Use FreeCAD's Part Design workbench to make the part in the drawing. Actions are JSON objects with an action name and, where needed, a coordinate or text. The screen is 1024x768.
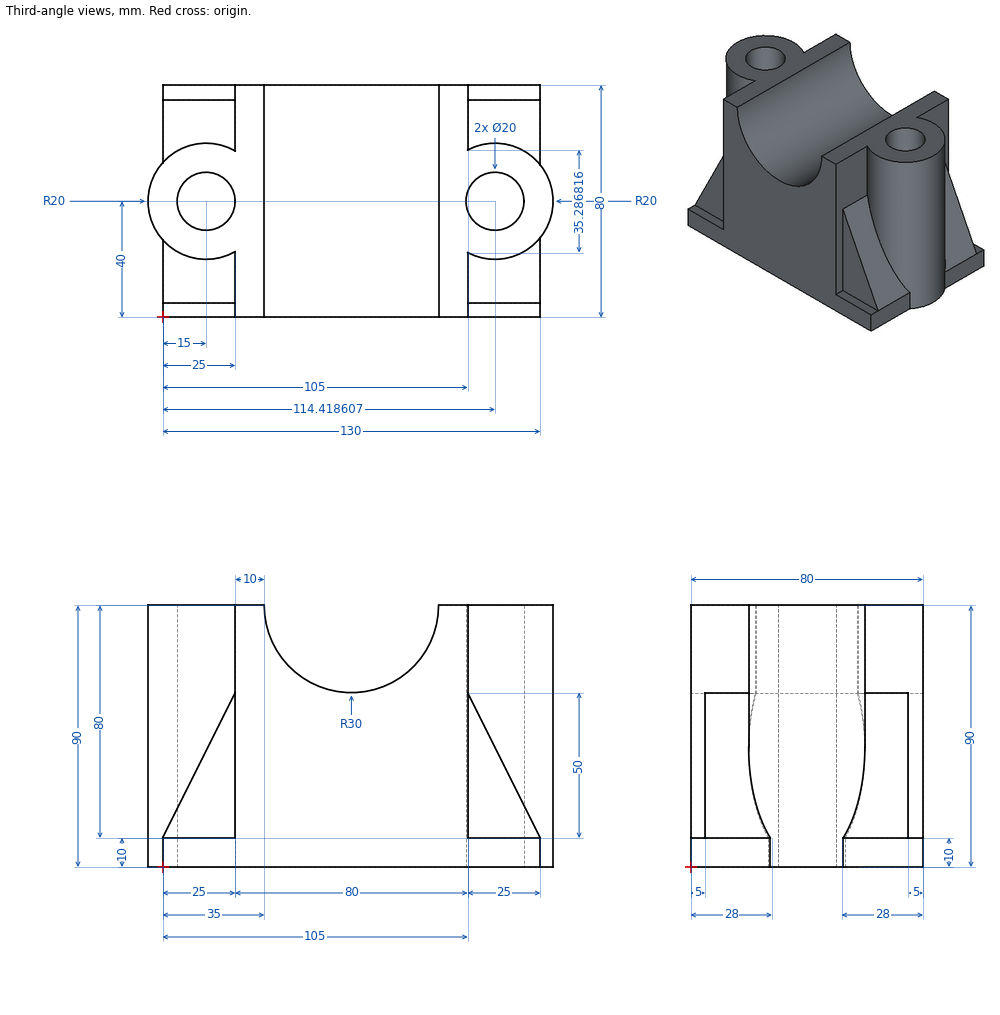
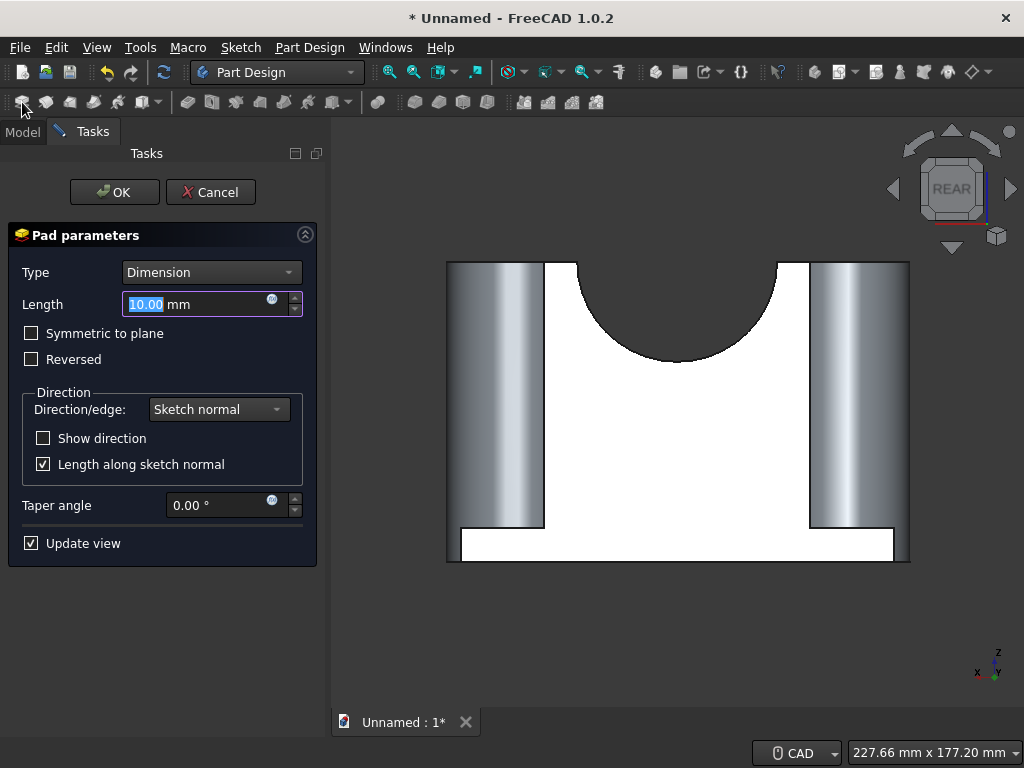
{"action": "type", "text": "28"}
{"action": "key", "text": "Tab"}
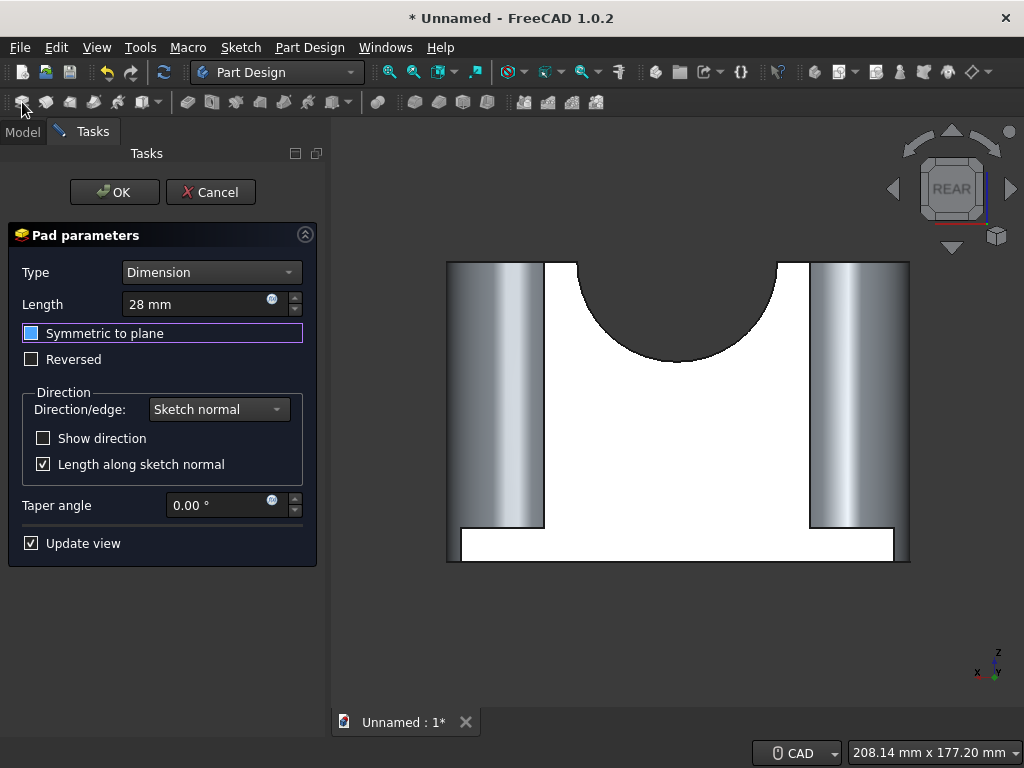
{"action": "left_click", "coordinate": [30, 359]}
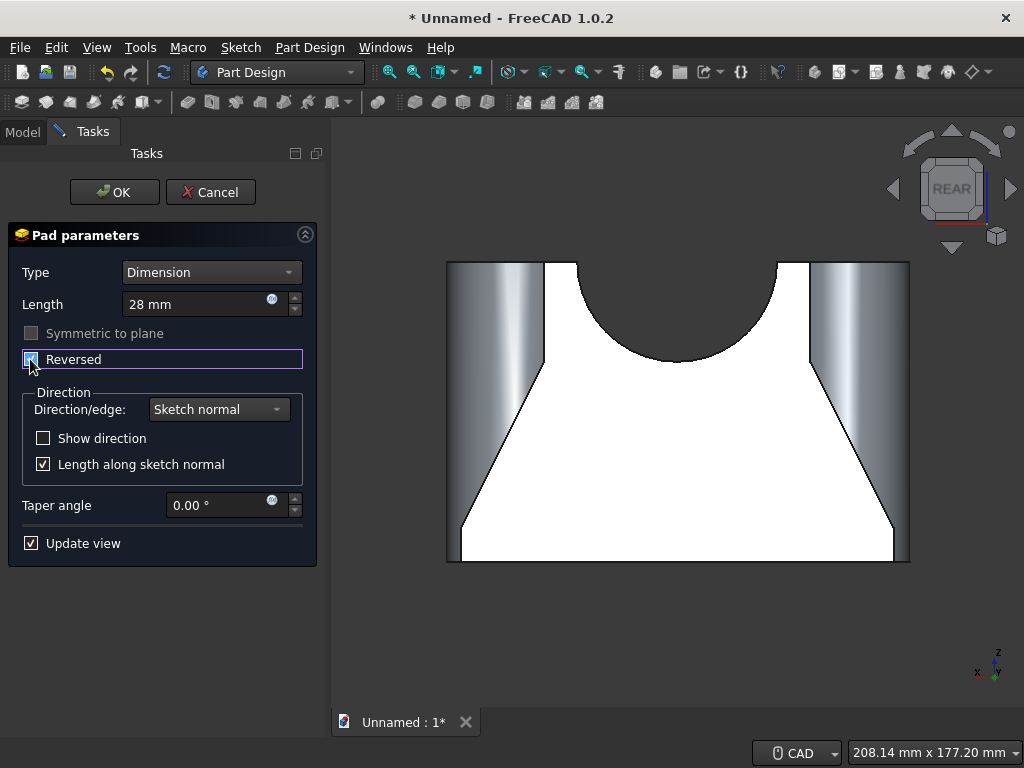
{"action": "left_click", "coordinate": [115, 192]}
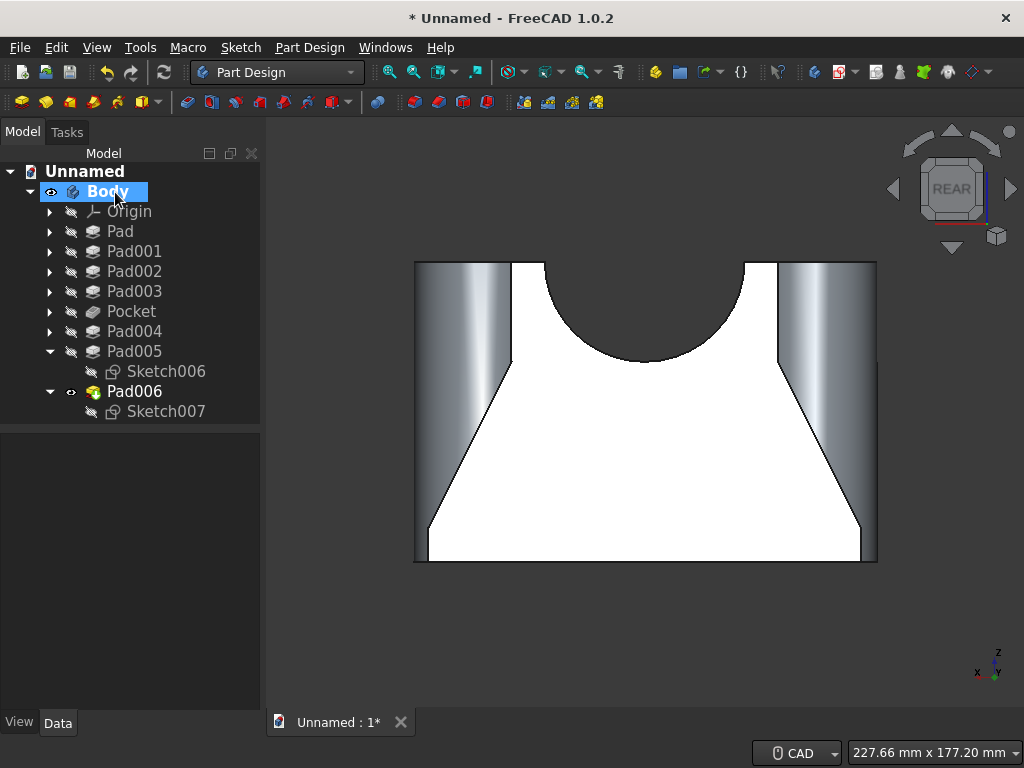
{"action": "left_click", "coordinate": [840, 72]}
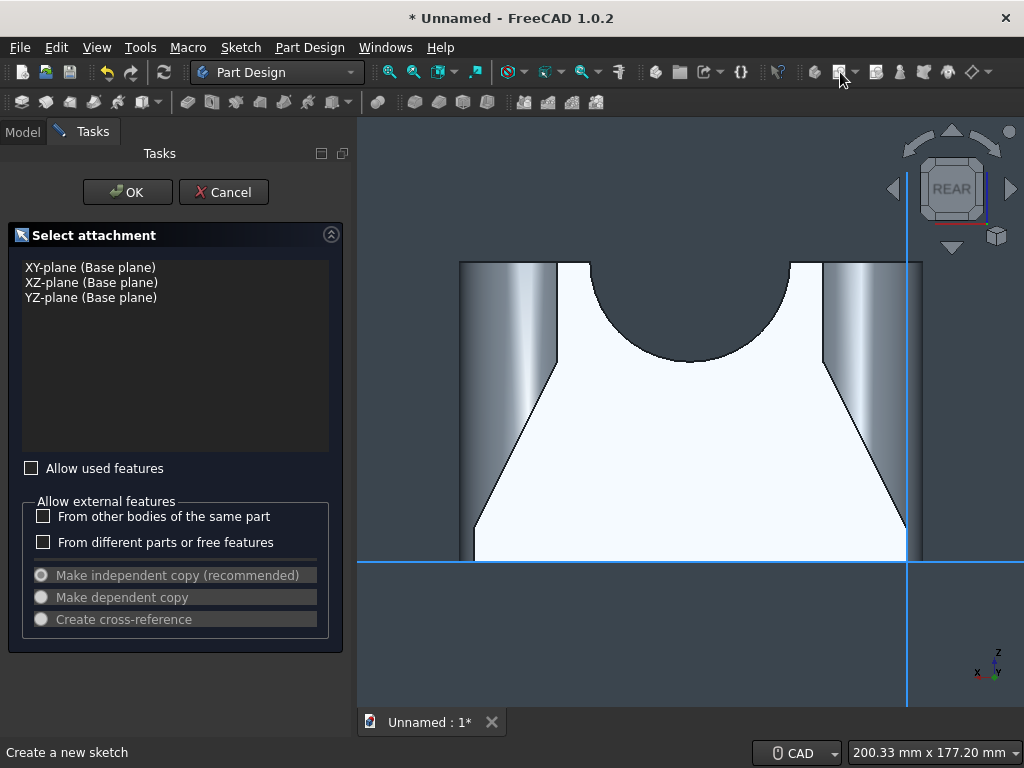
{"action": "left_click", "coordinate": [82, 282]}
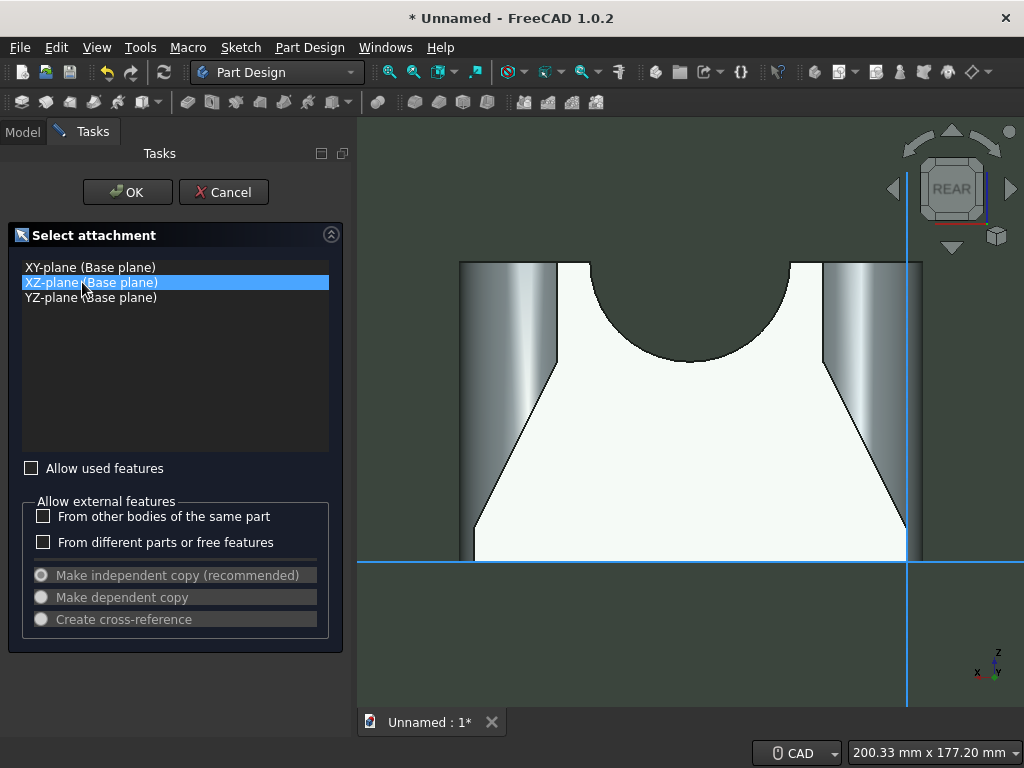
{"action": "left_click", "coordinate": [128, 192]}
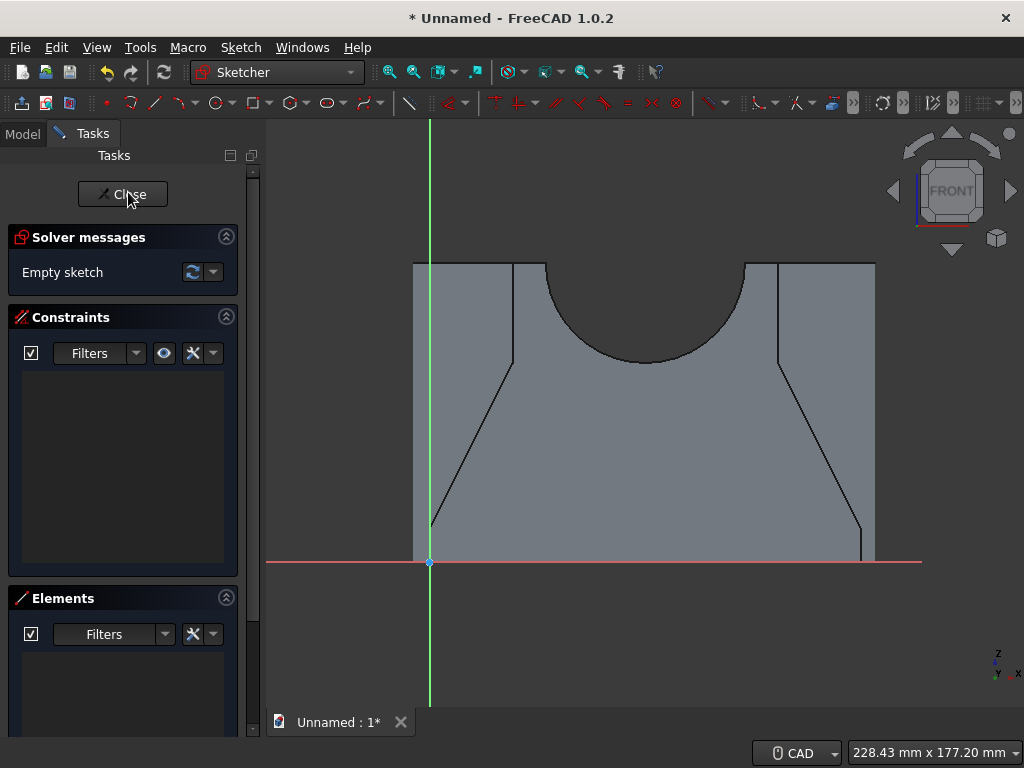
{"action": "scroll", "coordinate": [294, 189], "scroll_direction": "down", "scroll_amount": 1}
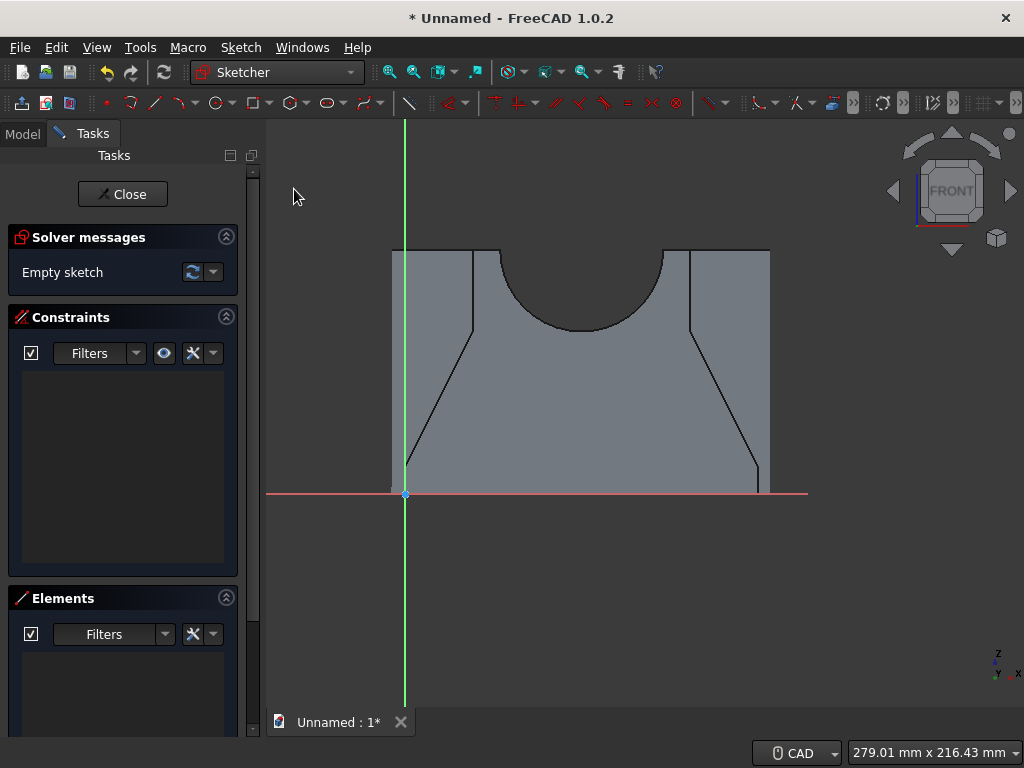
{"action": "left_click", "coordinate": [132, 104]}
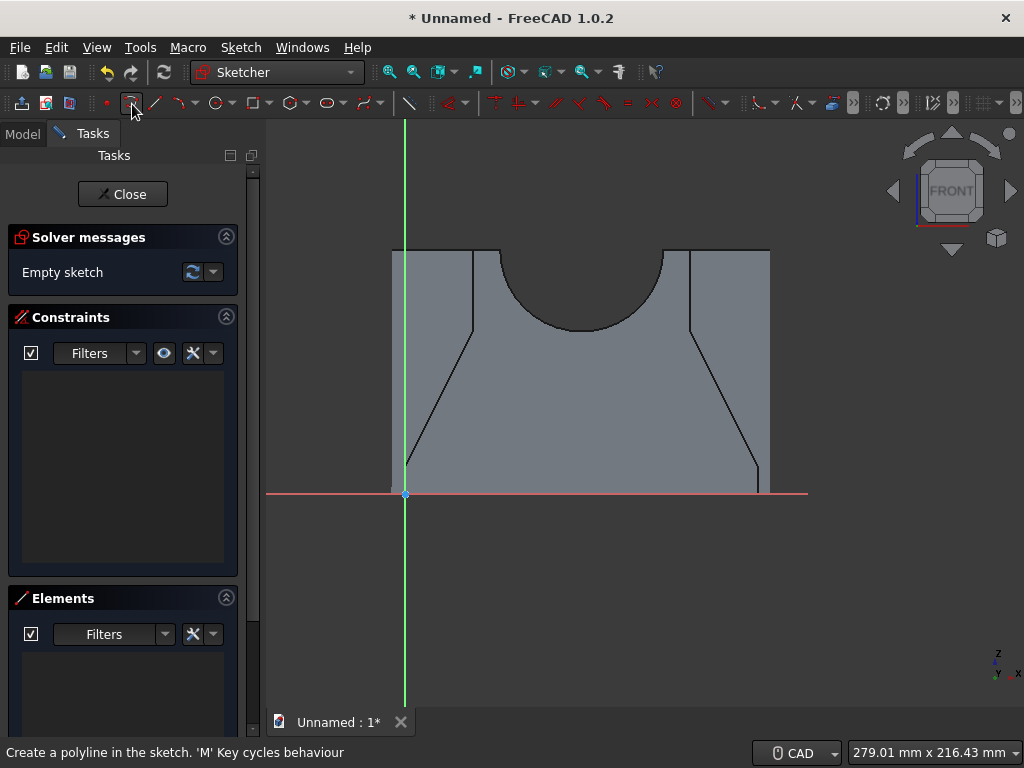
{"action": "left_click", "coordinate": [405, 467]}
{"action": "left_click", "coordinate": [473, 467]}
{"action": "left_click", "coordinate": [473, 331]}
{"action": "left_click", "coordinate": [405, 468]}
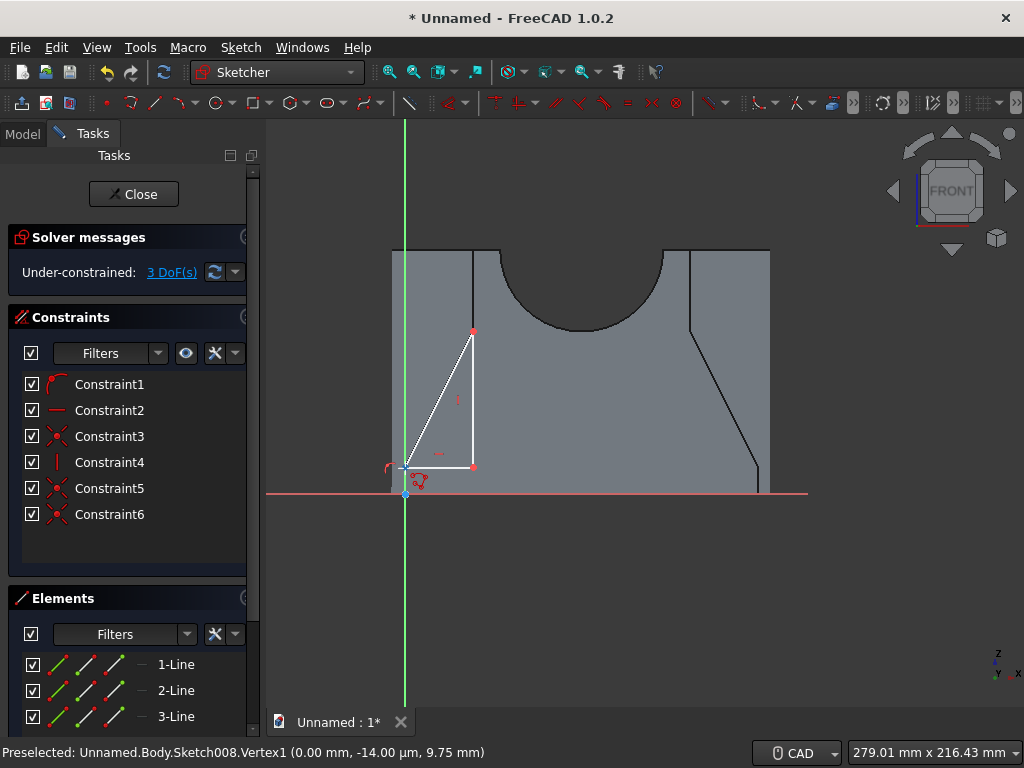
{"action": "left_click", "coordinate": [690, 467]}
{"action": "left_click", "coordinate": [758, 467]}
{"action": "left_click", "coordinate": [690, 331]}
{"action": "left_click", "coordinate": [690, 468]}
{"action": "key", "text": "Escape"}
{"action": "key", "text": "Escape"}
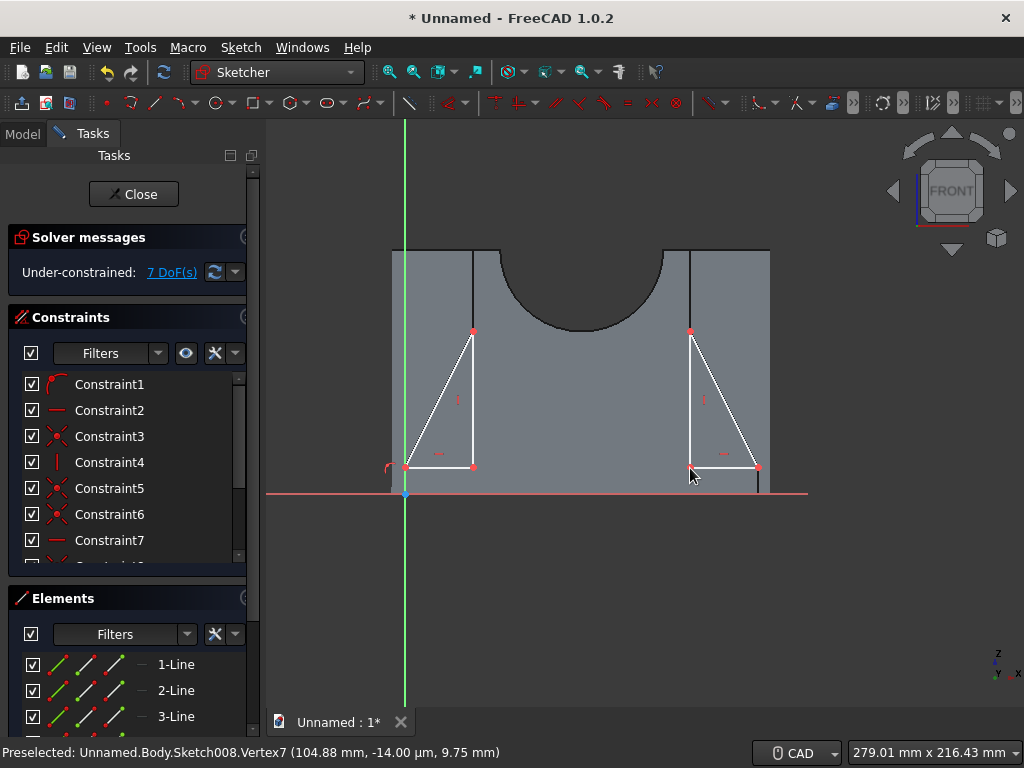
{"action": "left_click", "coordinate": [448, 104]}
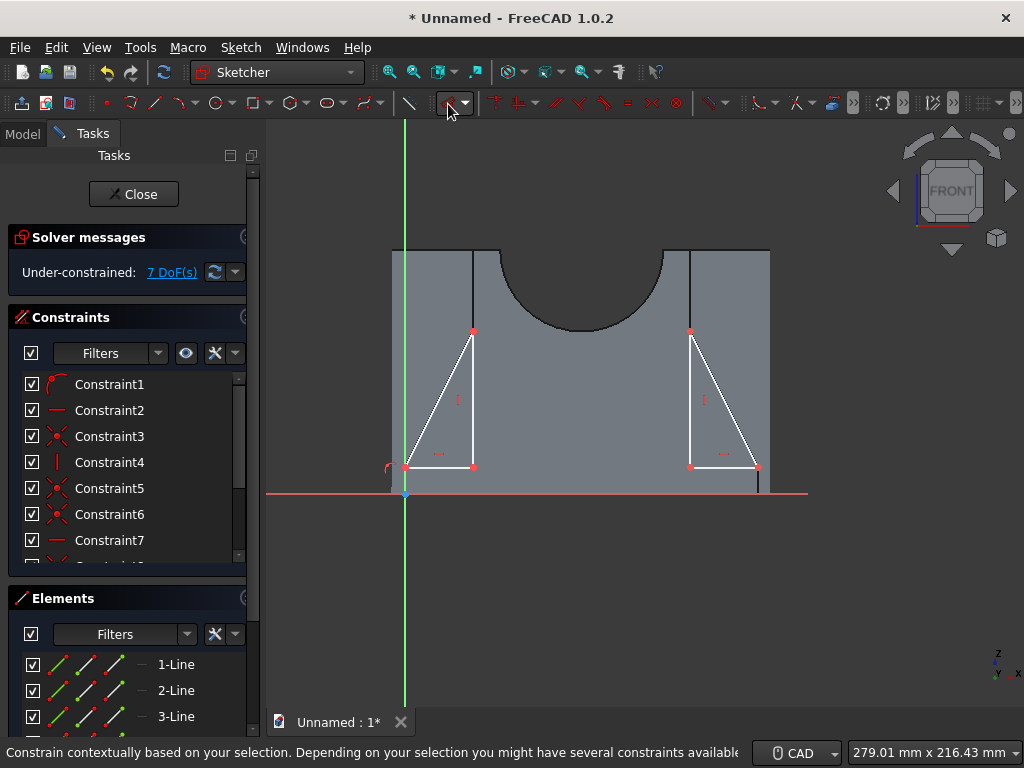
{"action": "left_click", "coordinate": [425, 468]}
{"action": "left_click", "coordinate": [439, 434]}